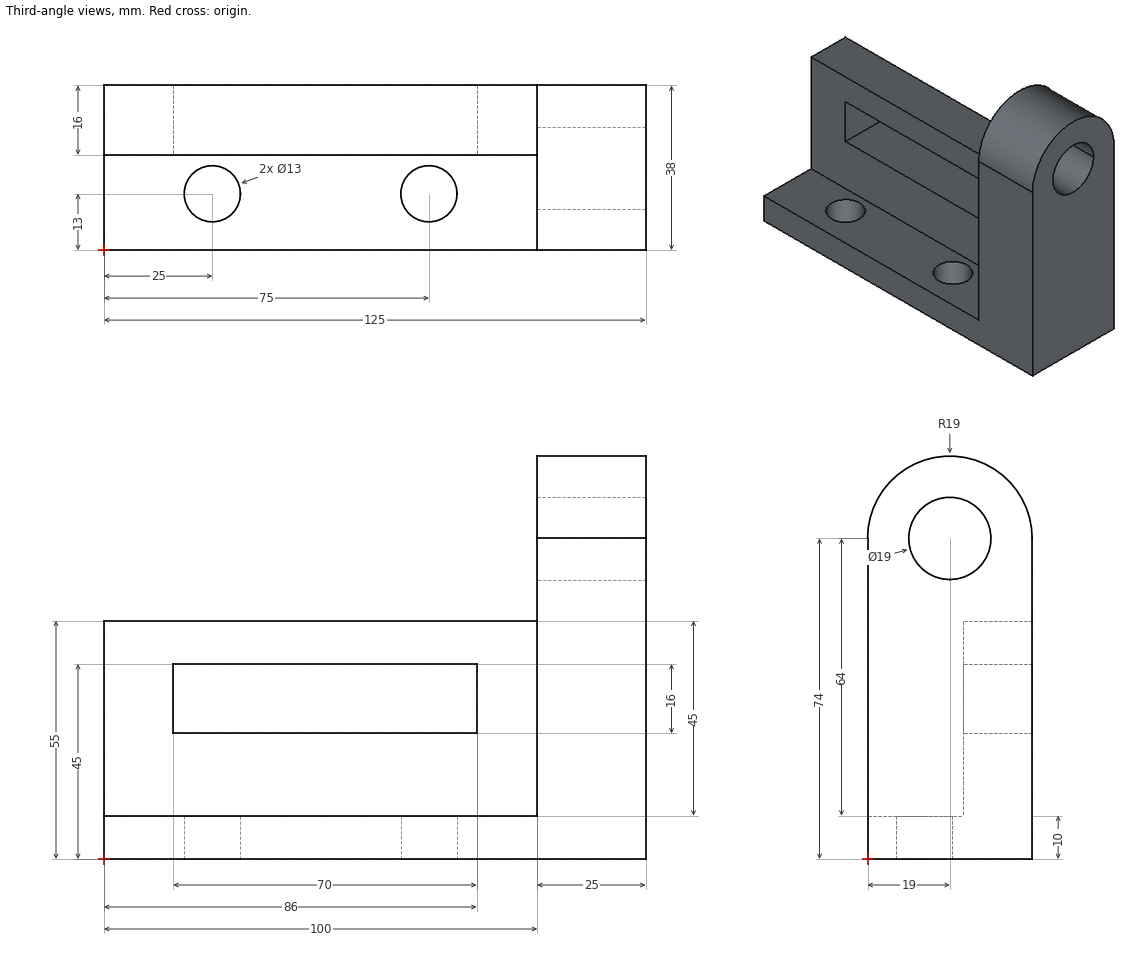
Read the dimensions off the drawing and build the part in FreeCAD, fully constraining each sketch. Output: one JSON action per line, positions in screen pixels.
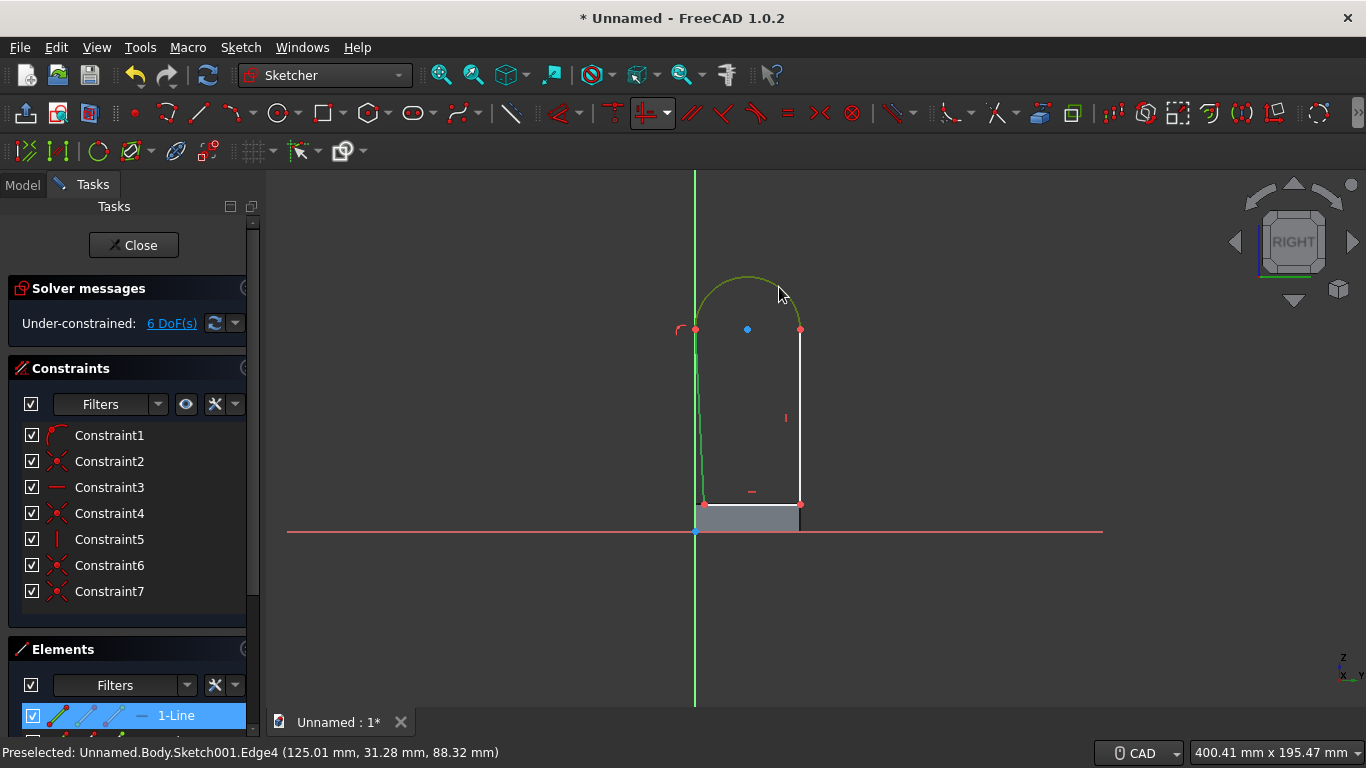
{"action": "left_click", "coordinate": [756, 114]}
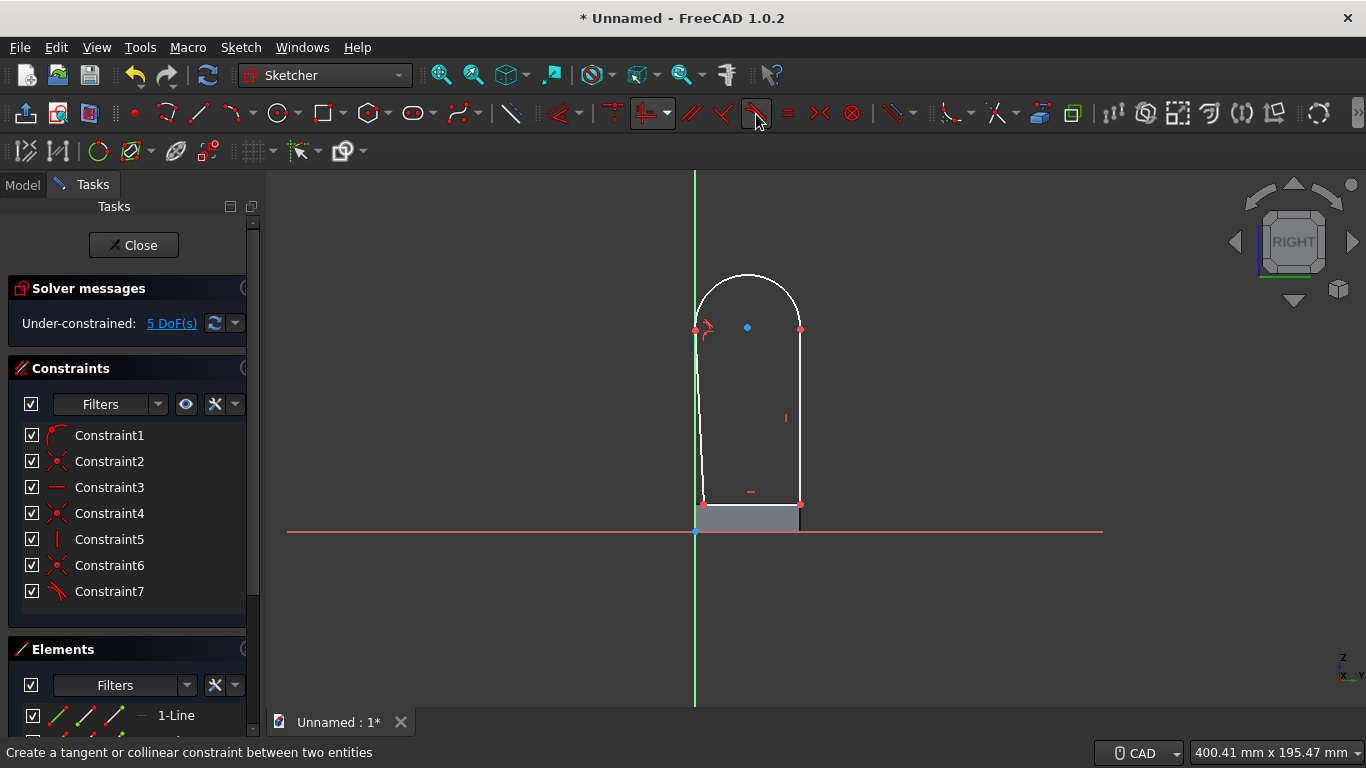
{"action": "left_click", "coordinate": [800, 453]}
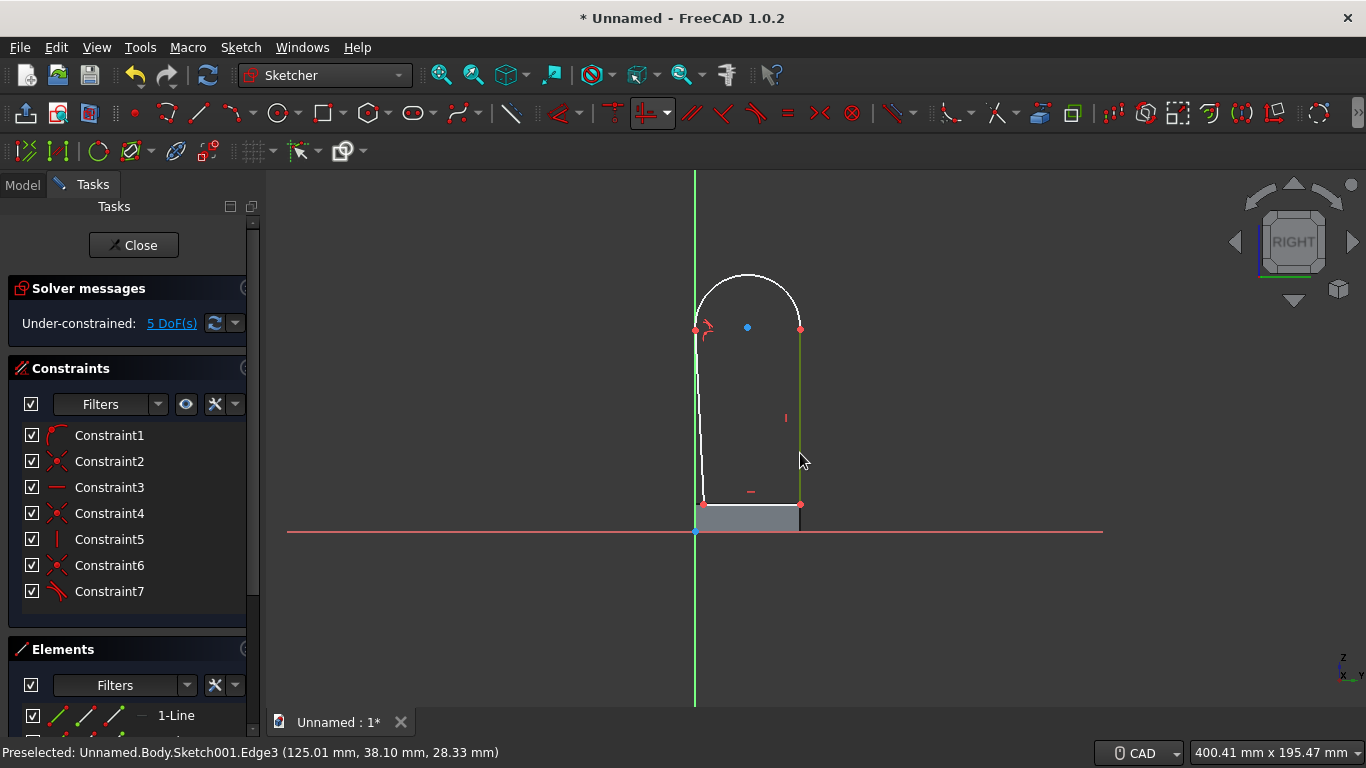
{"action": "left_click", "coordinate": [779, 286]}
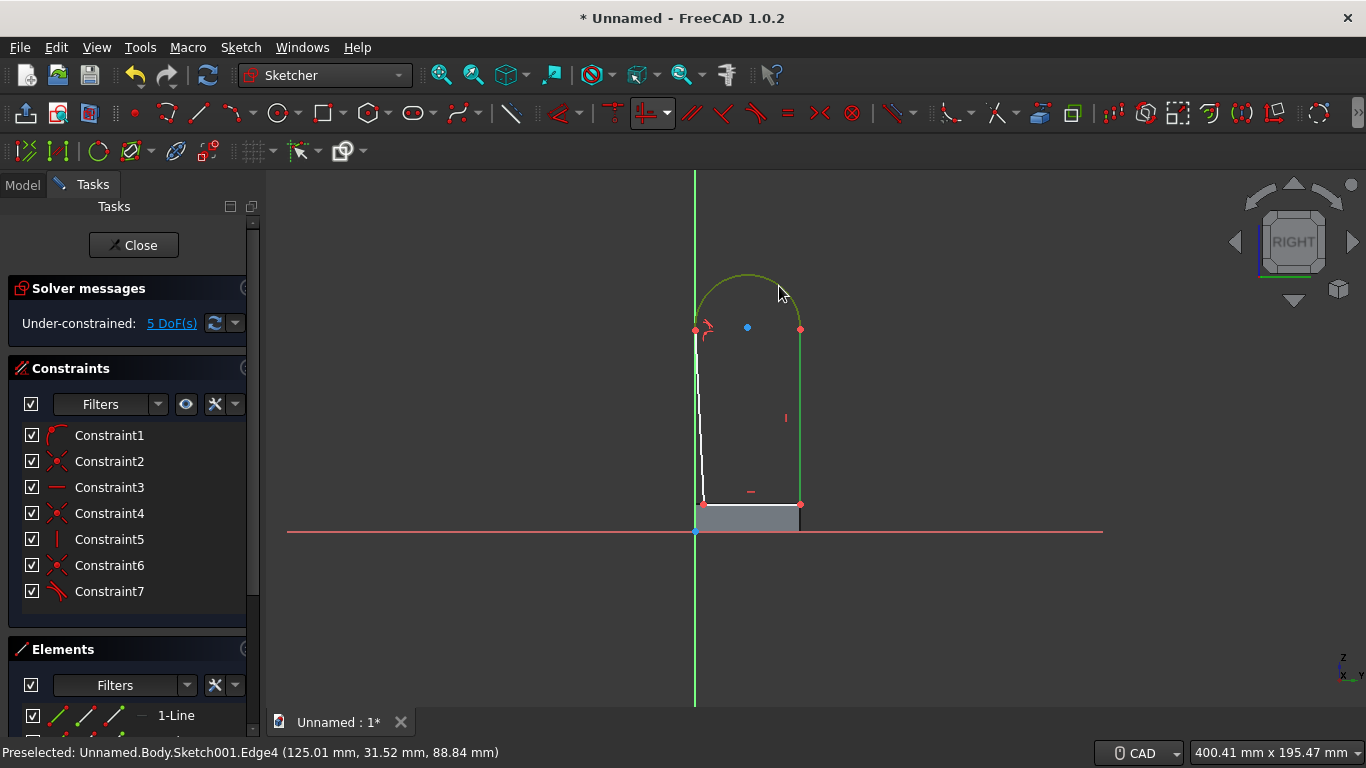
{"action": "left_click", "coordinate": [756, 114]}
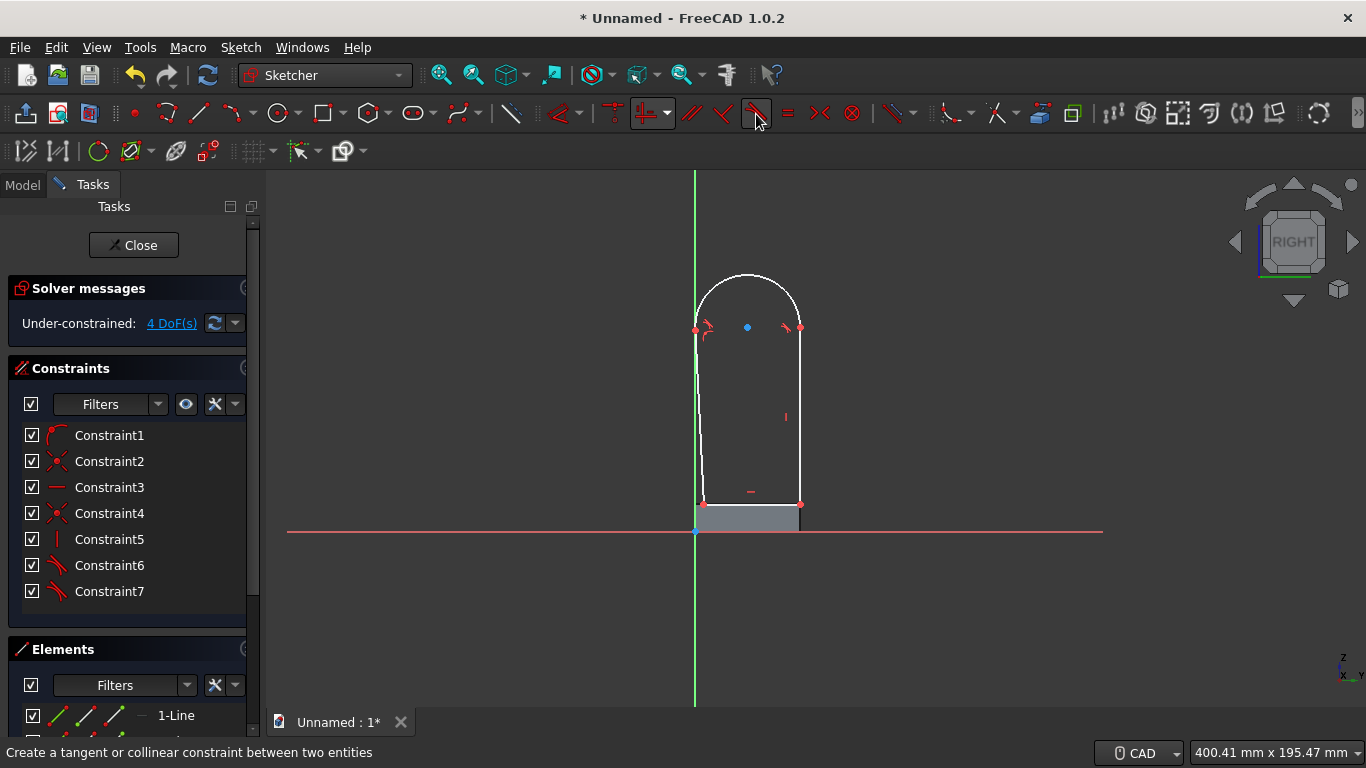
{"action": "left_click", "coordinate": [698, 383]}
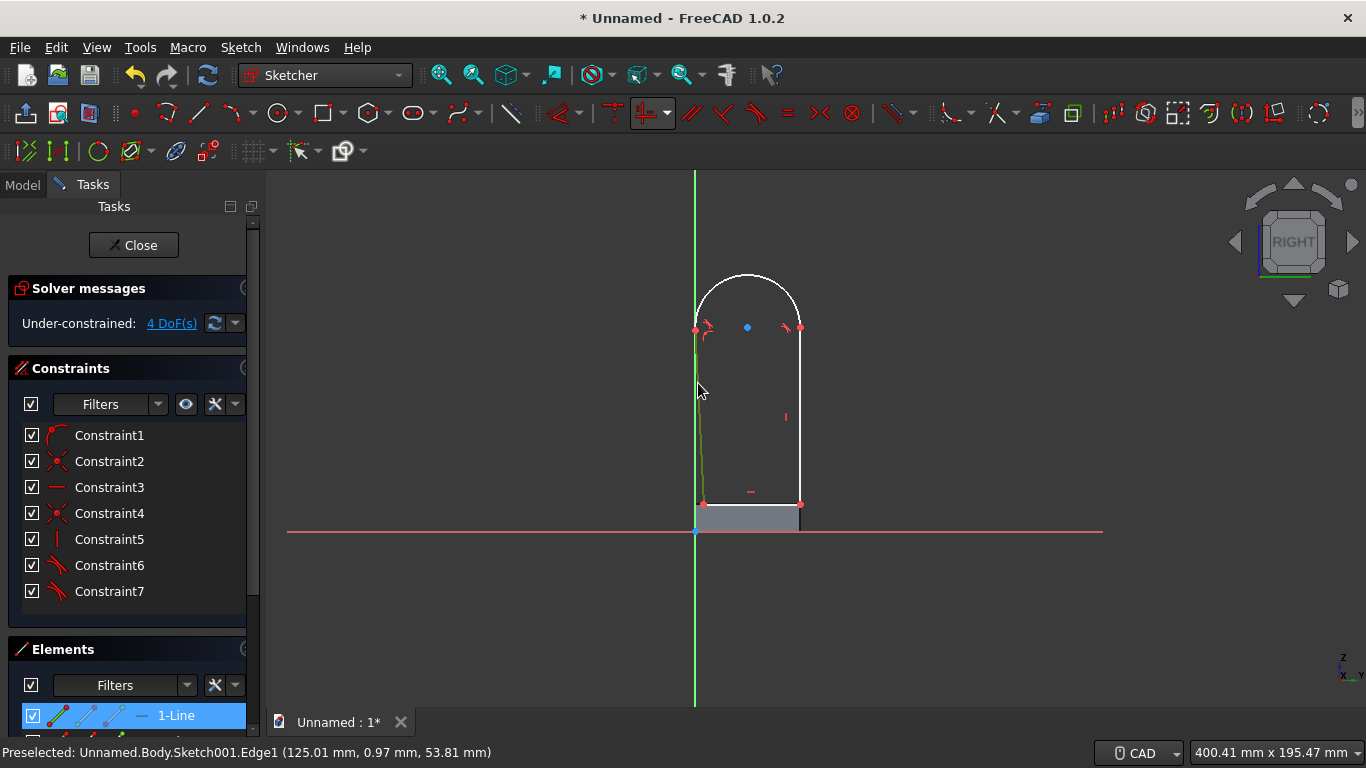
{"action": "left_click", "coordinate": [670, 114]}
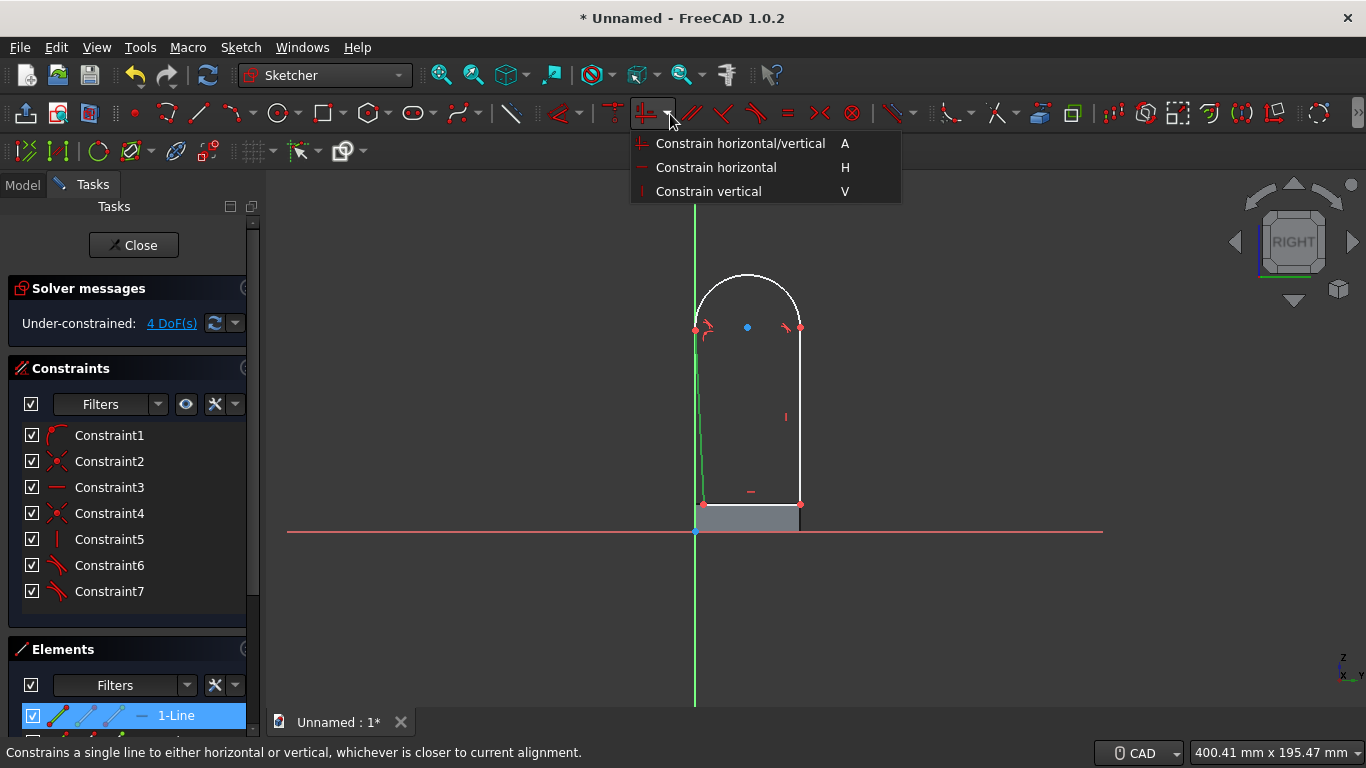
{"action": "left_click", "coordinate": [766, 191]}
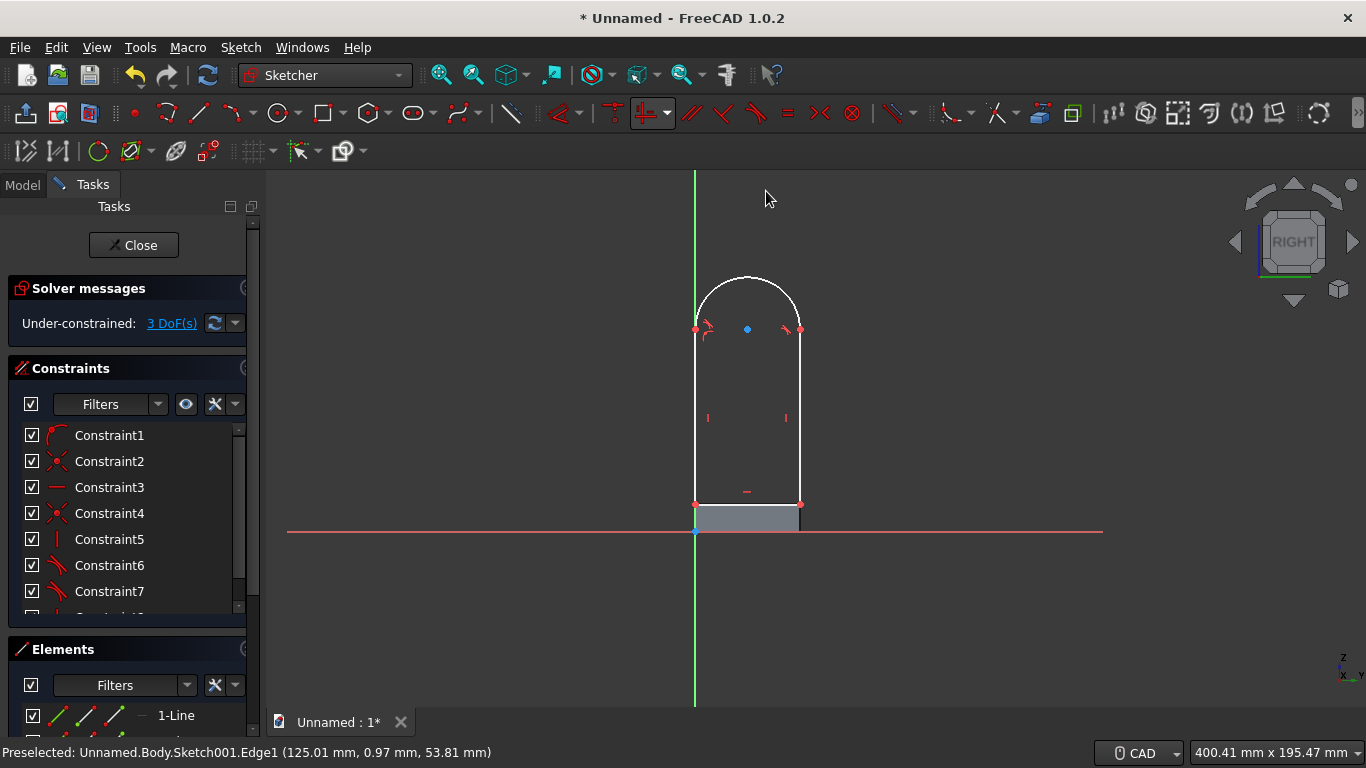
{"action": "left_click", "coordinate": [558, 114]}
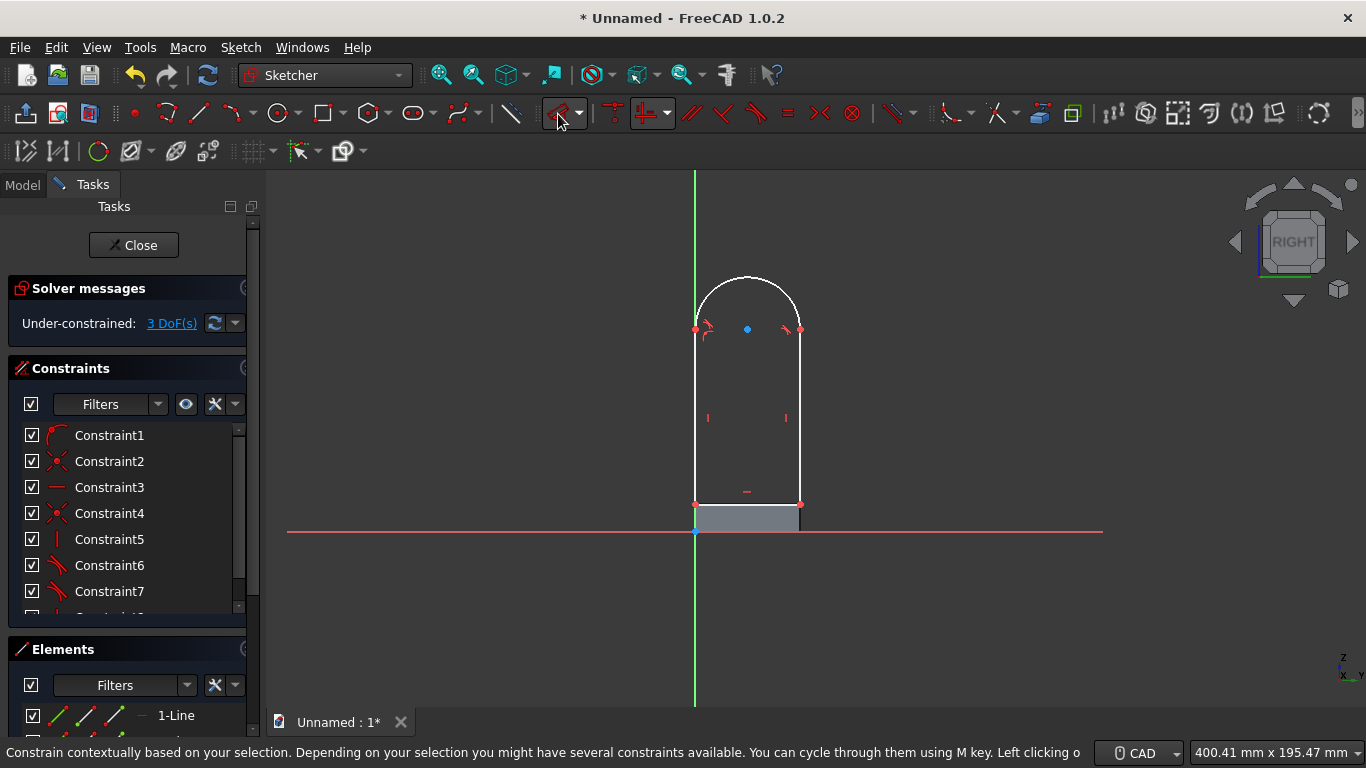
{"action": "left_click", "coordinate": [778, 287]}
{"action": "left_click", "coordinate": [797, 261]}